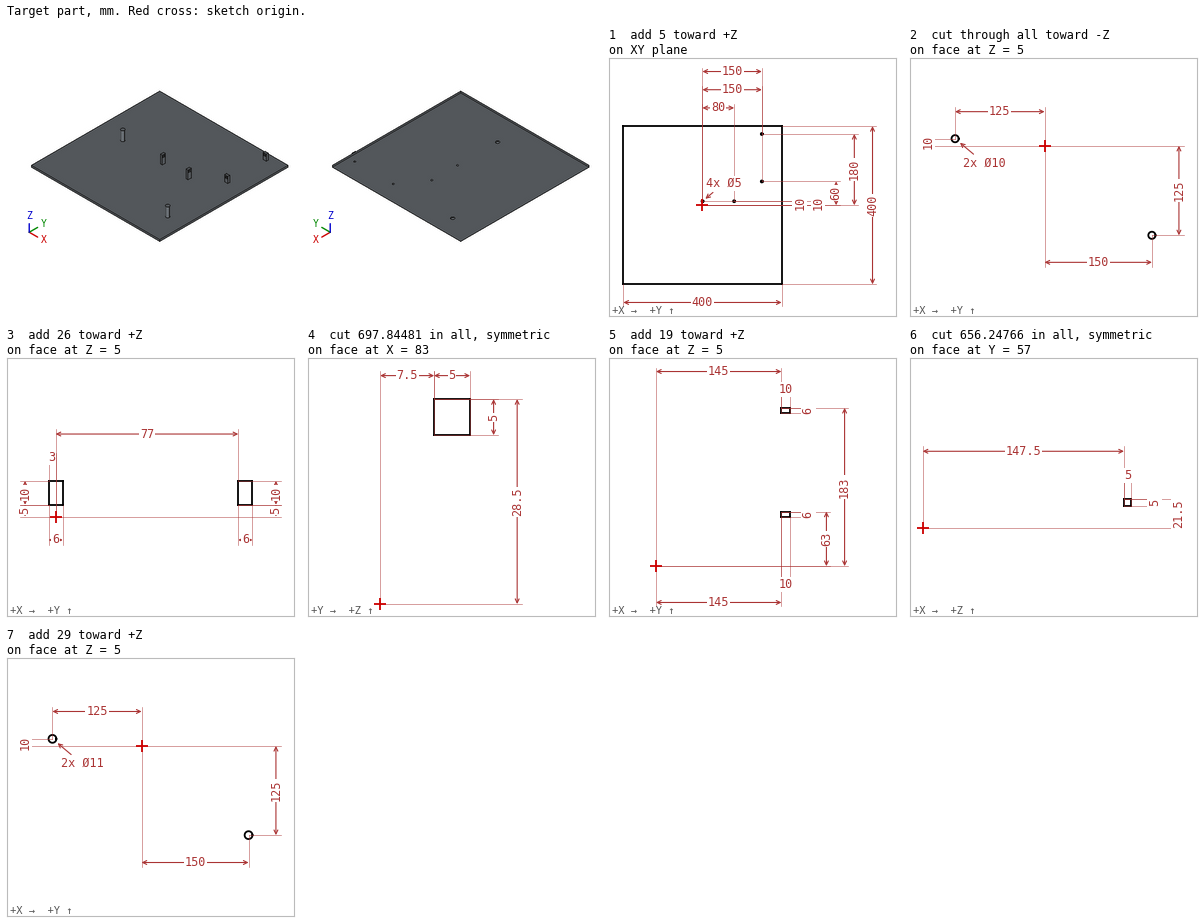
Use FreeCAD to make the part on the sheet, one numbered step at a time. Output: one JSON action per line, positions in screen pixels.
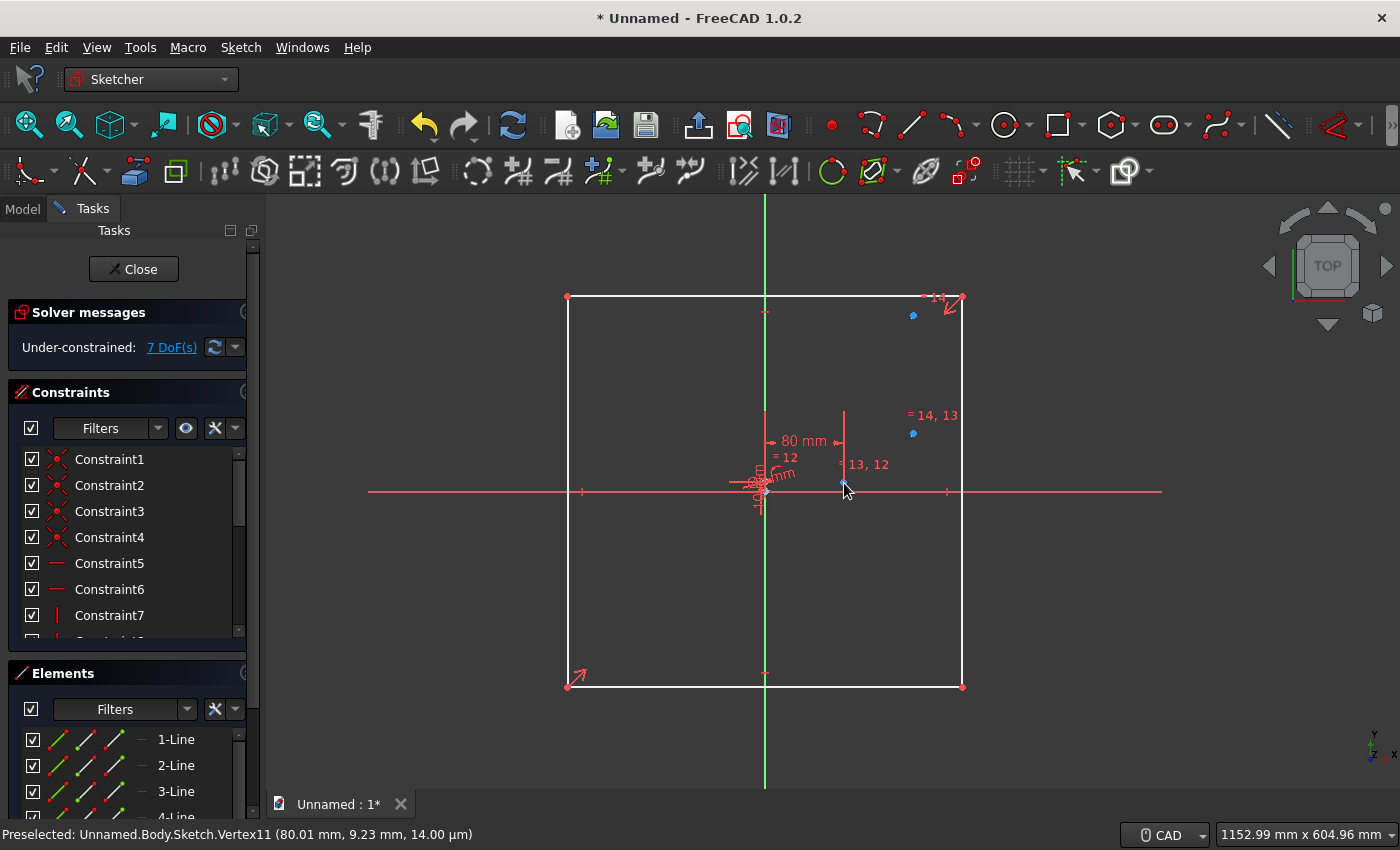
{"action": "scroll", "coordinate": [844, 483], "scroll_direction": "up", "scroll_amount": 7}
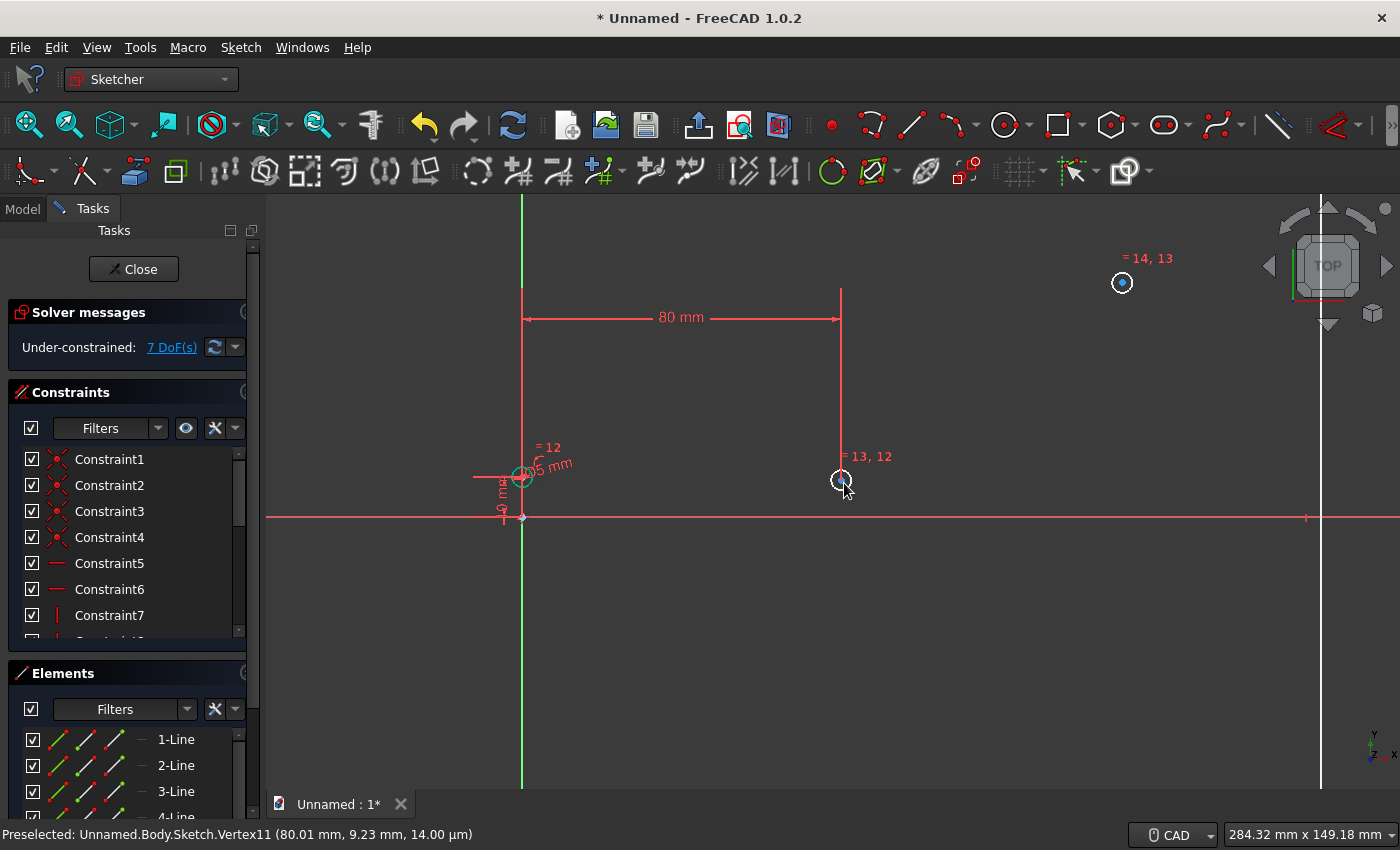
{"action": "left_click", "coordinate": [841, 480]}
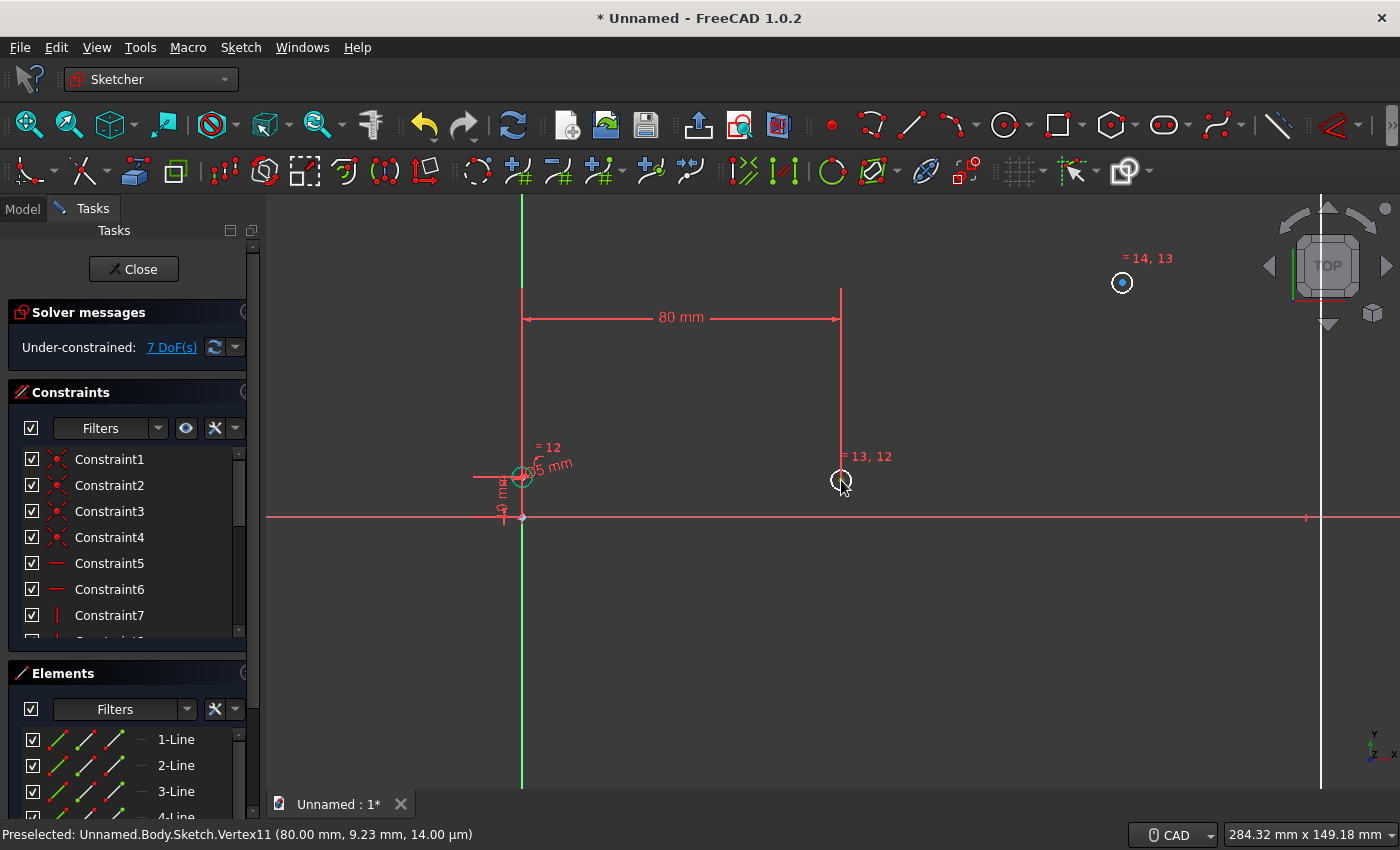
{"action": "key", "text": "i"}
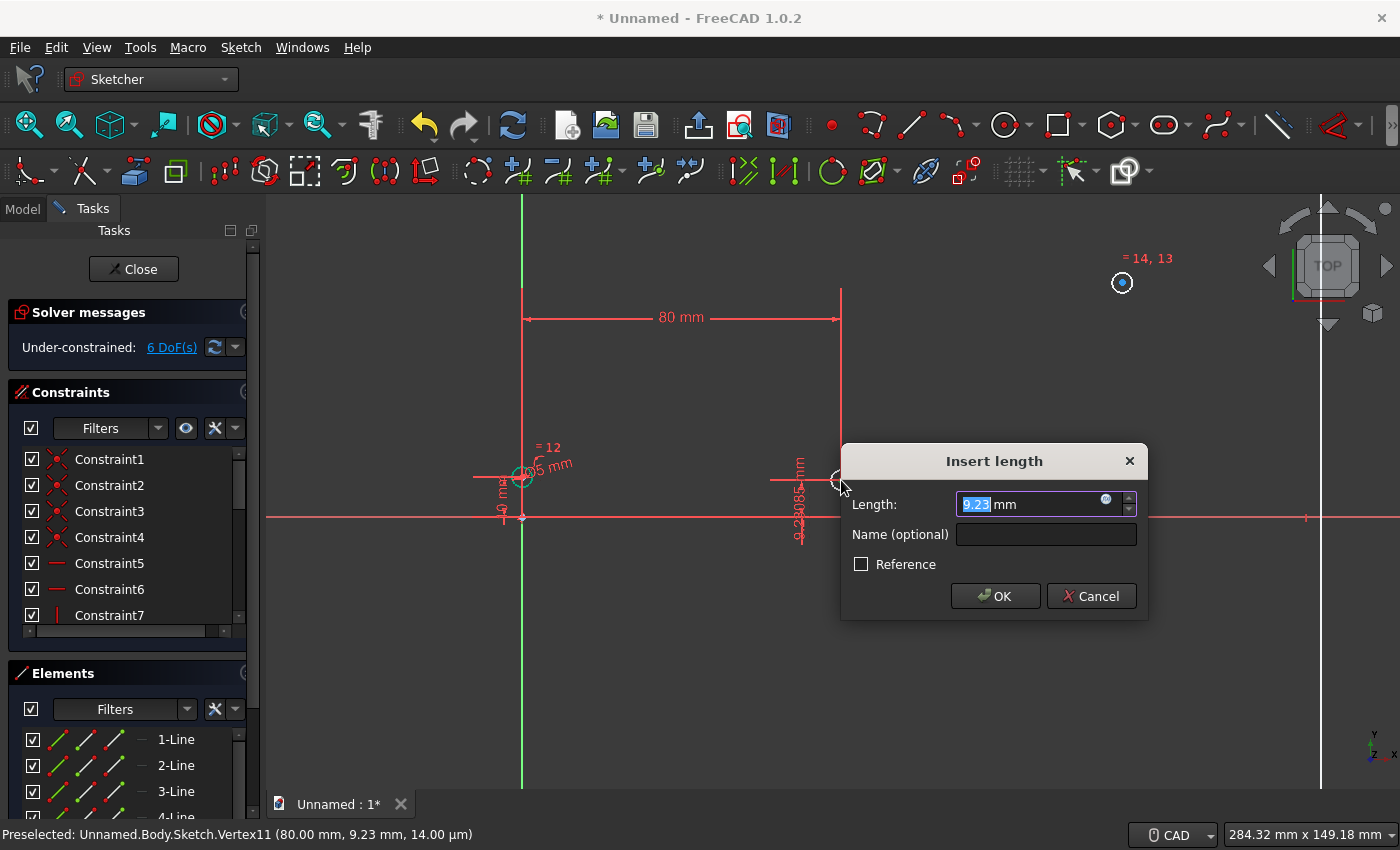
{"action": "type", "text": "10"}
{"action": "key", "text": "Return"}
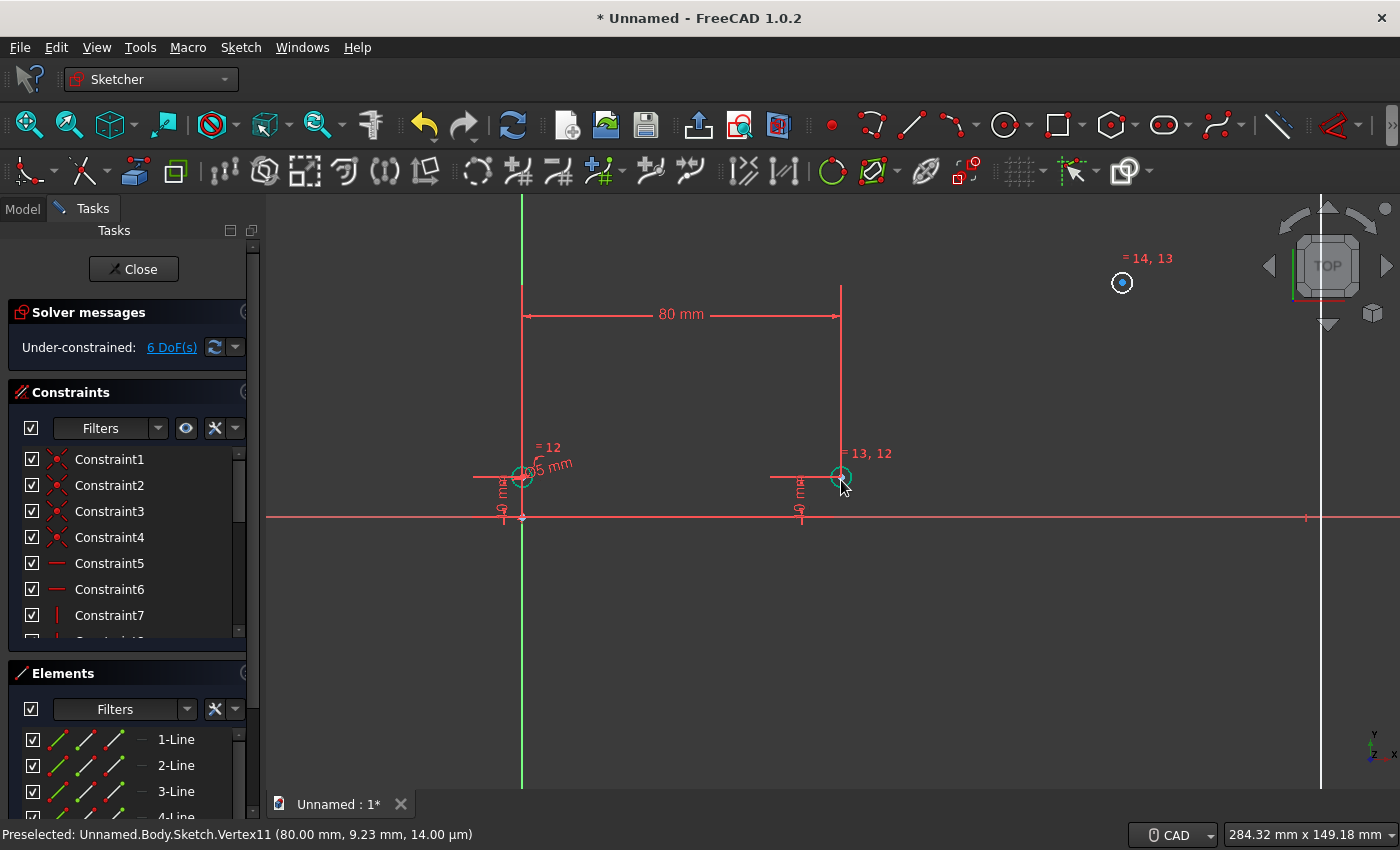
{"action": "scroll", "coordinate": [844, 483], "scroll_direction": "down", "scroll_amount": 7}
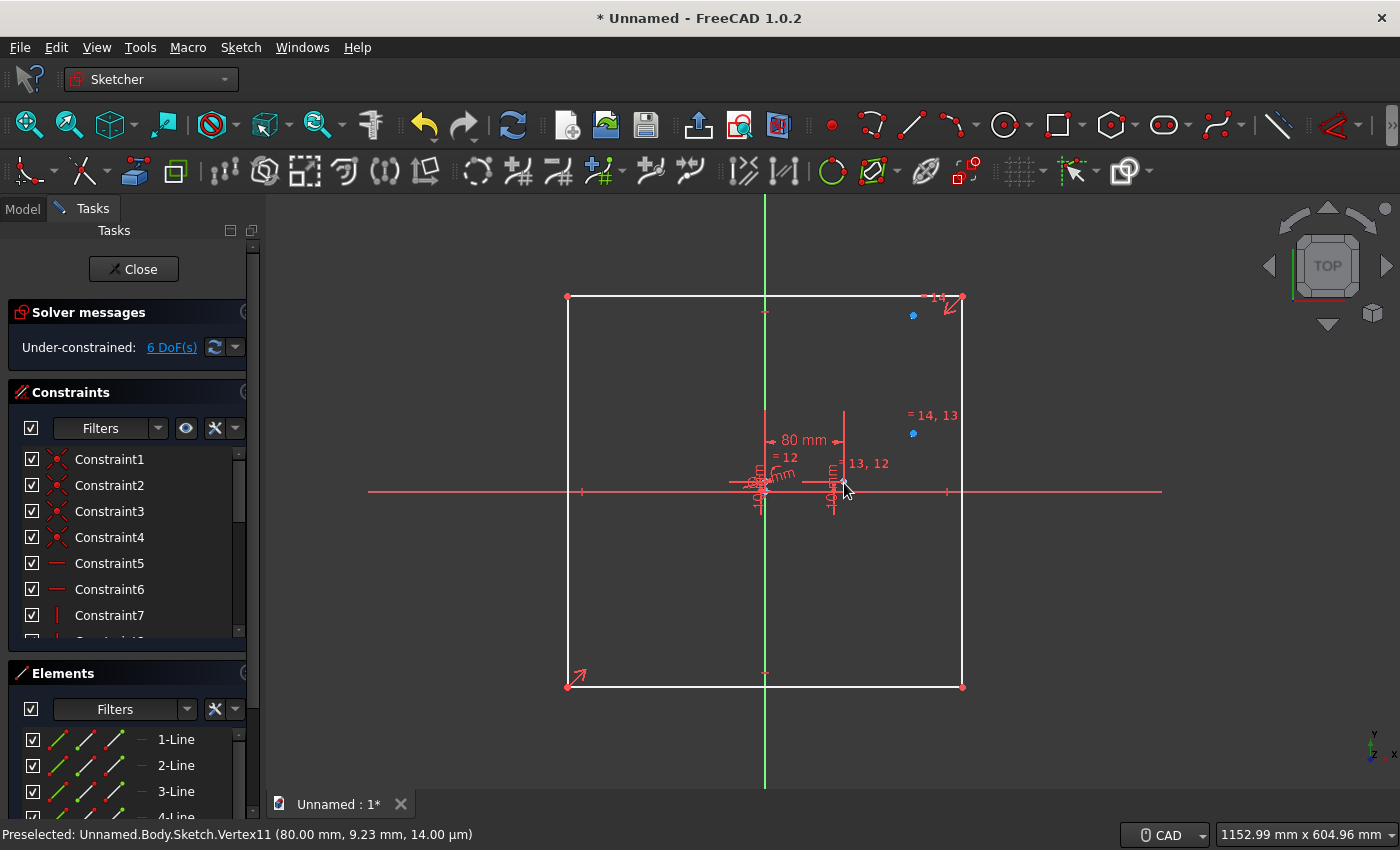
{"action": "left_click", "coordinate": [913, 434]}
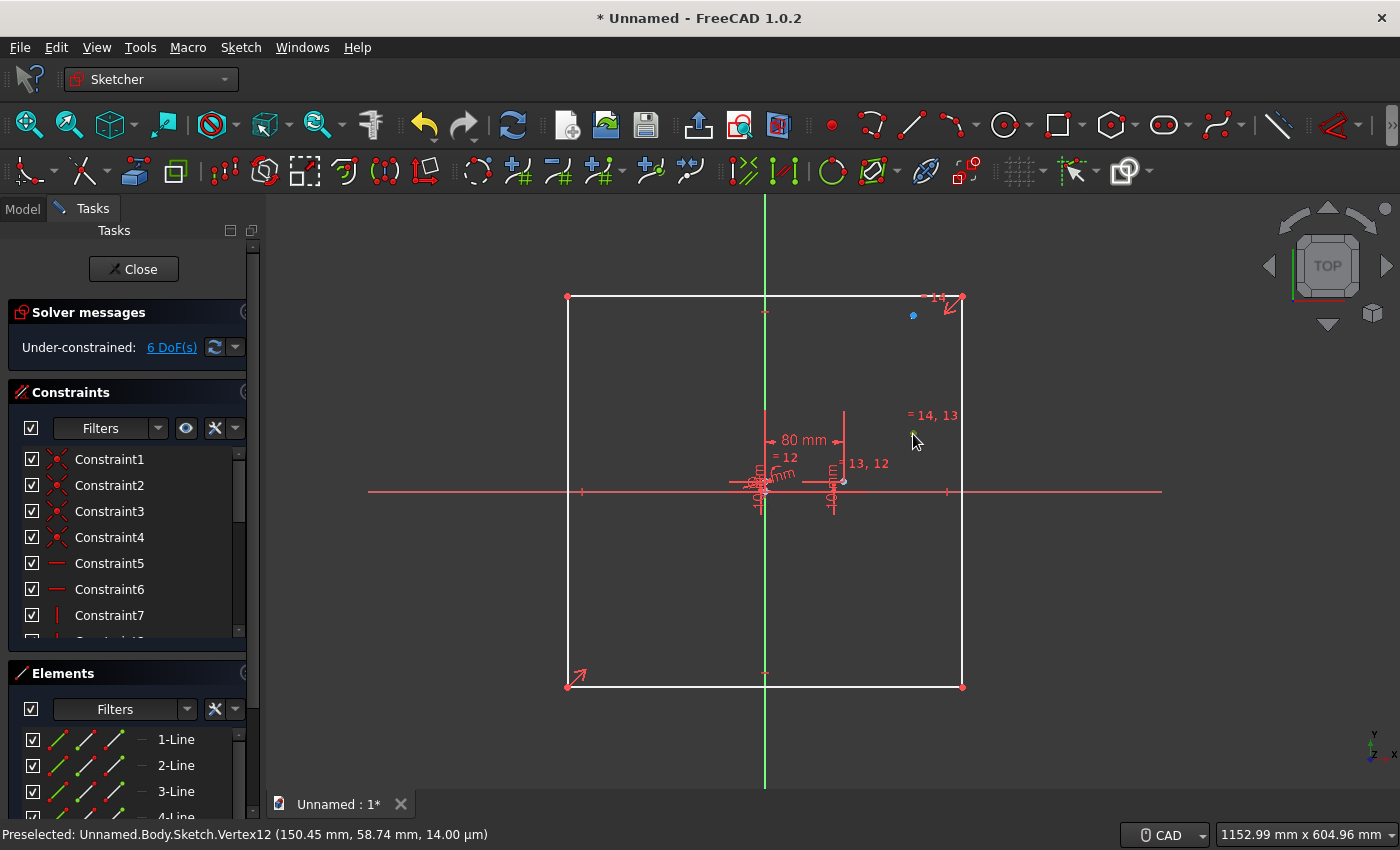
{"action": "left_click", "coordinate": [1360, 126]}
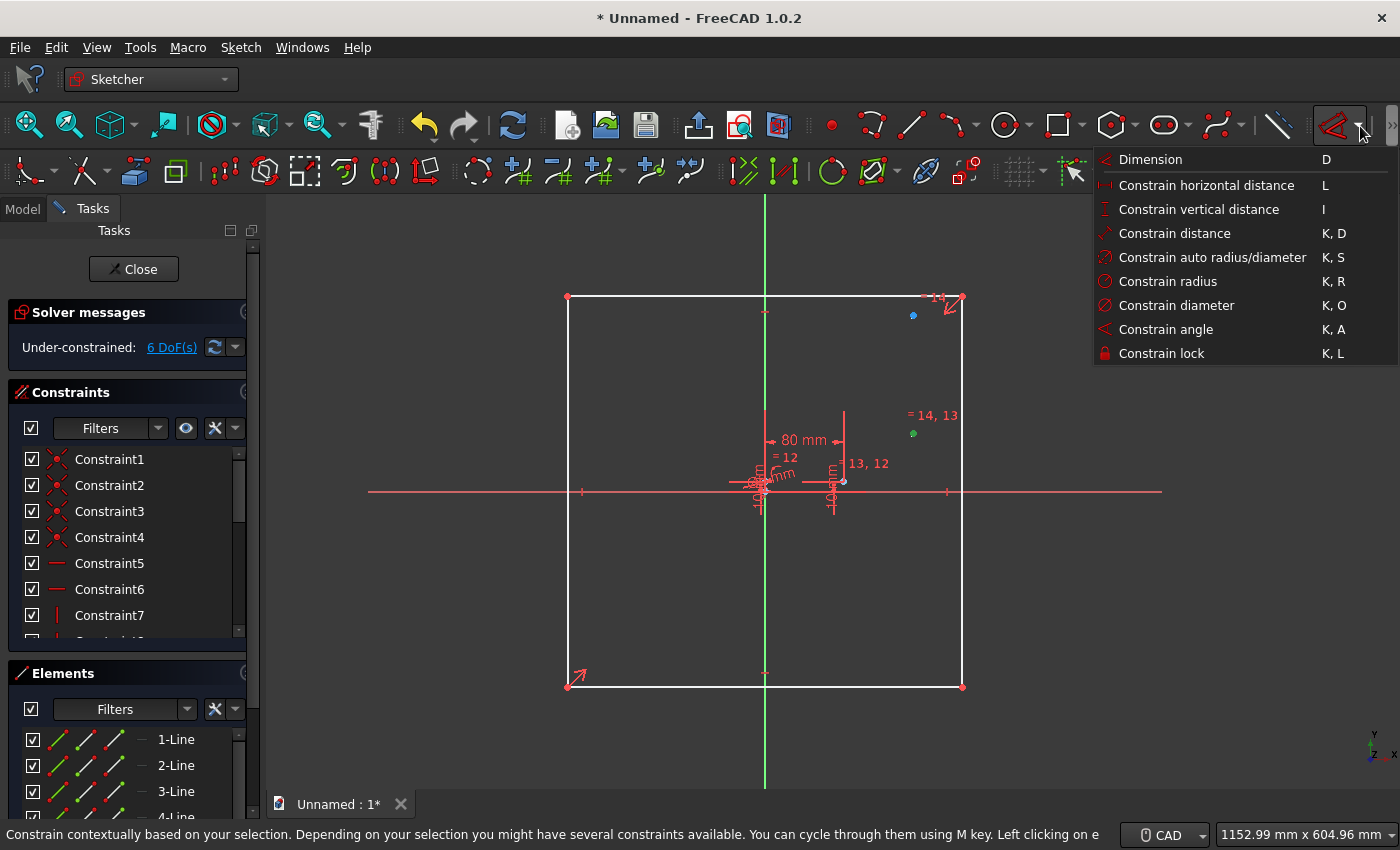
{"action": "left_click", "coordinate": [1246, 209]}